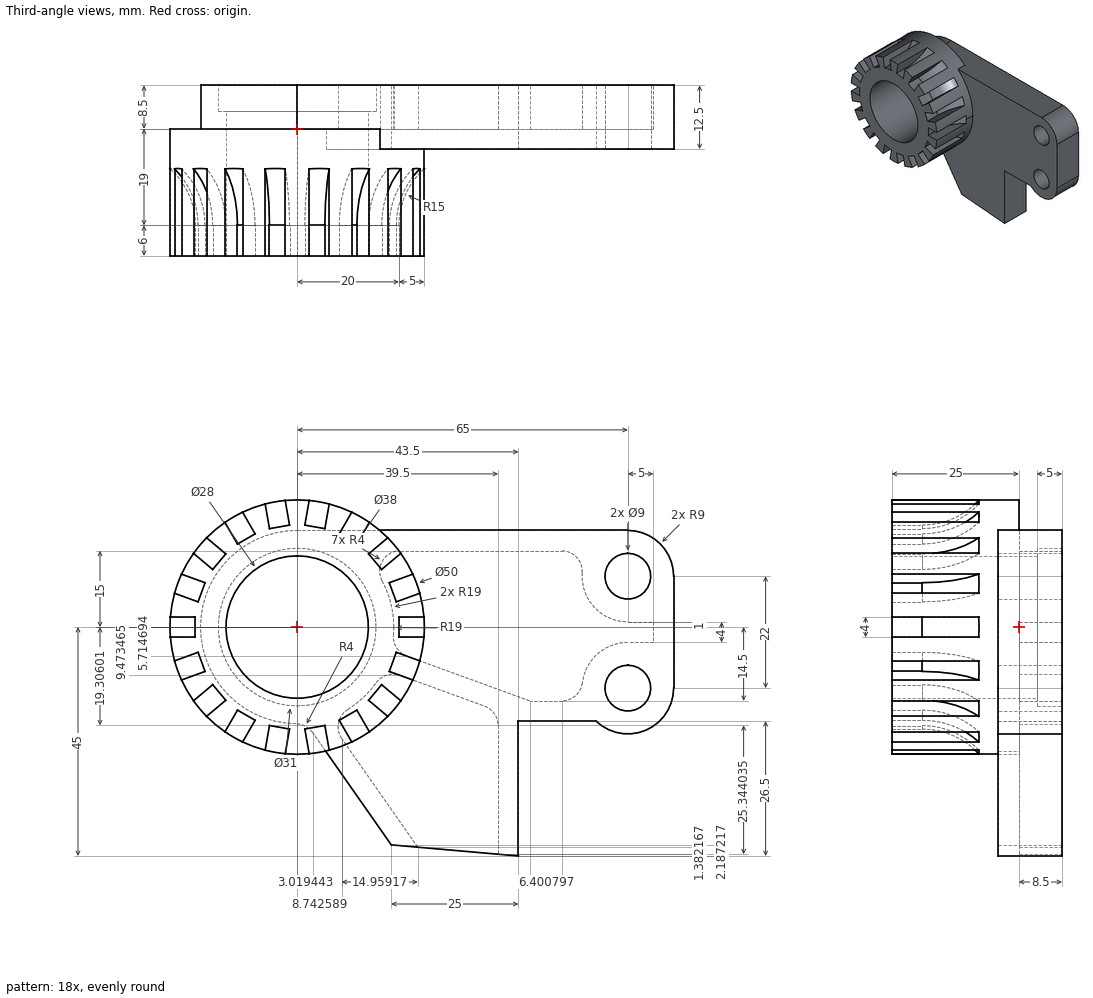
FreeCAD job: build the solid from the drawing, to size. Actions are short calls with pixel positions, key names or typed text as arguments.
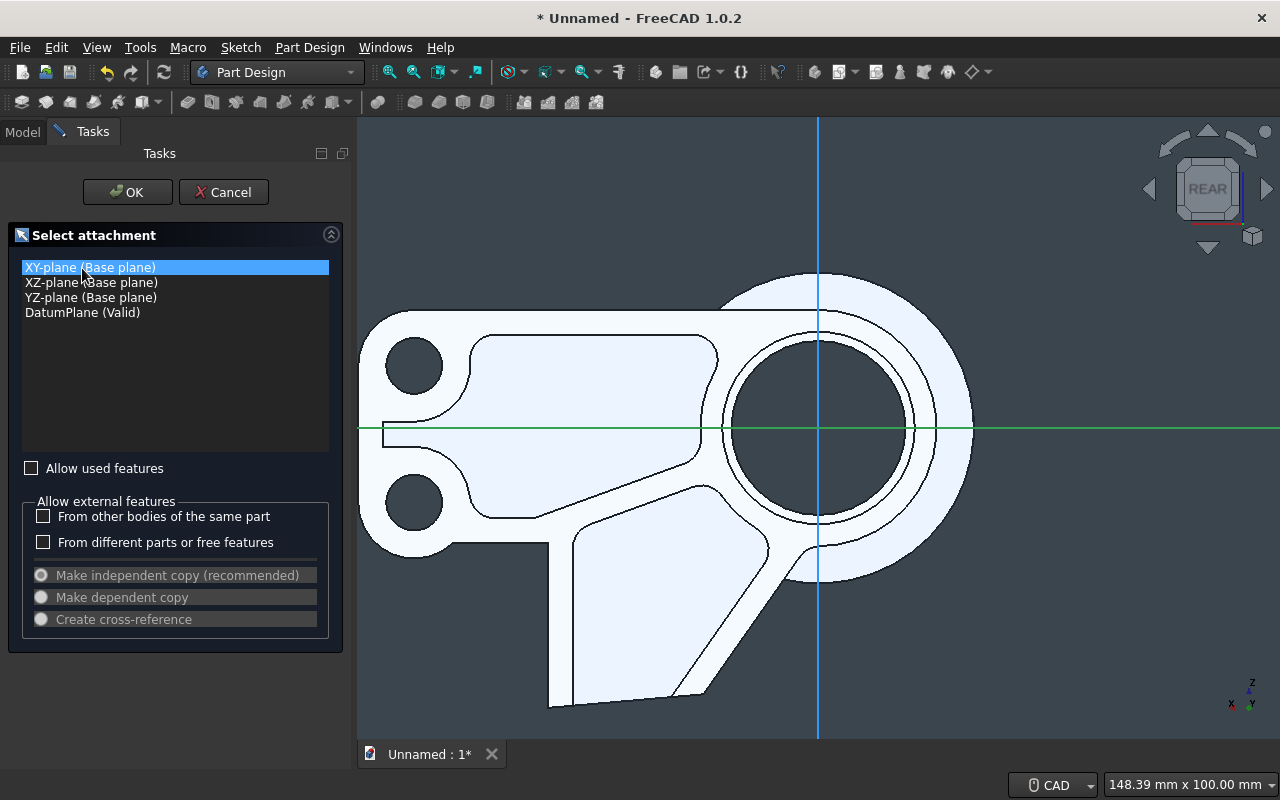
click(128, 192)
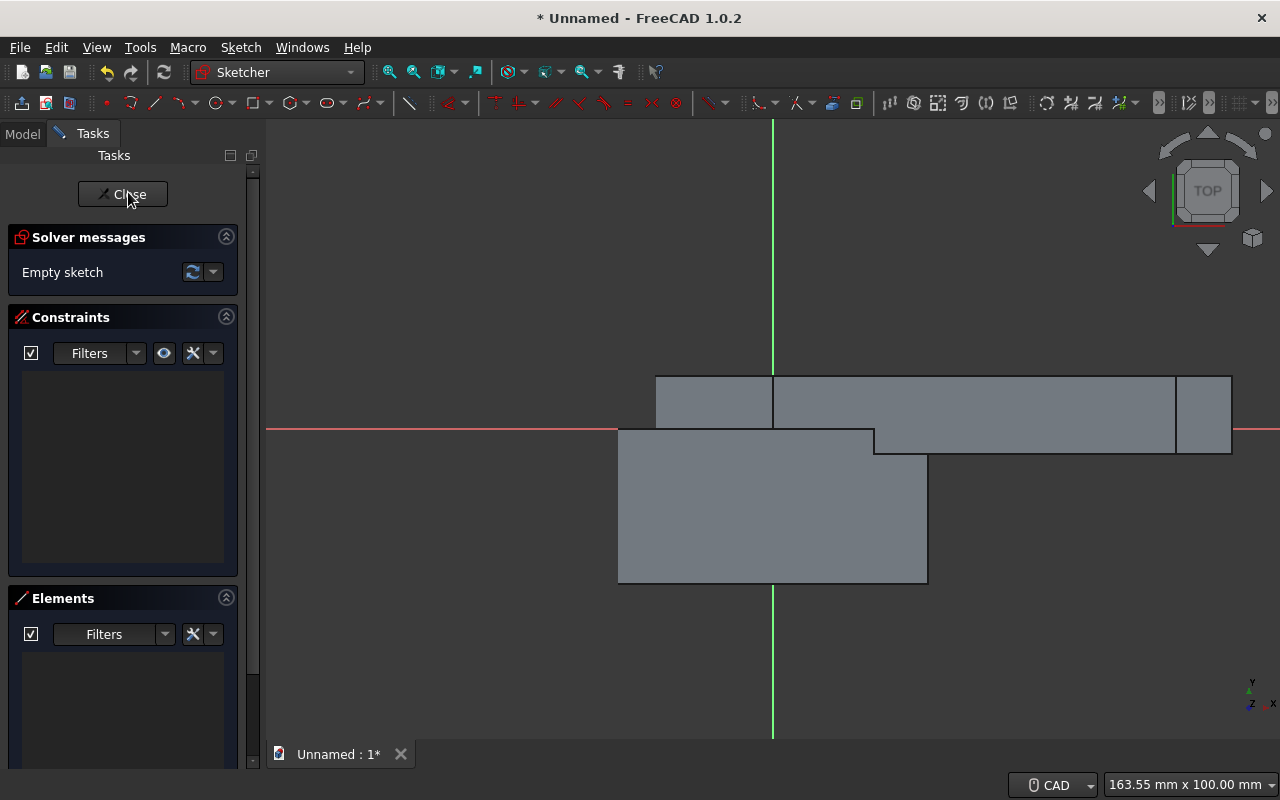
click(70, 104)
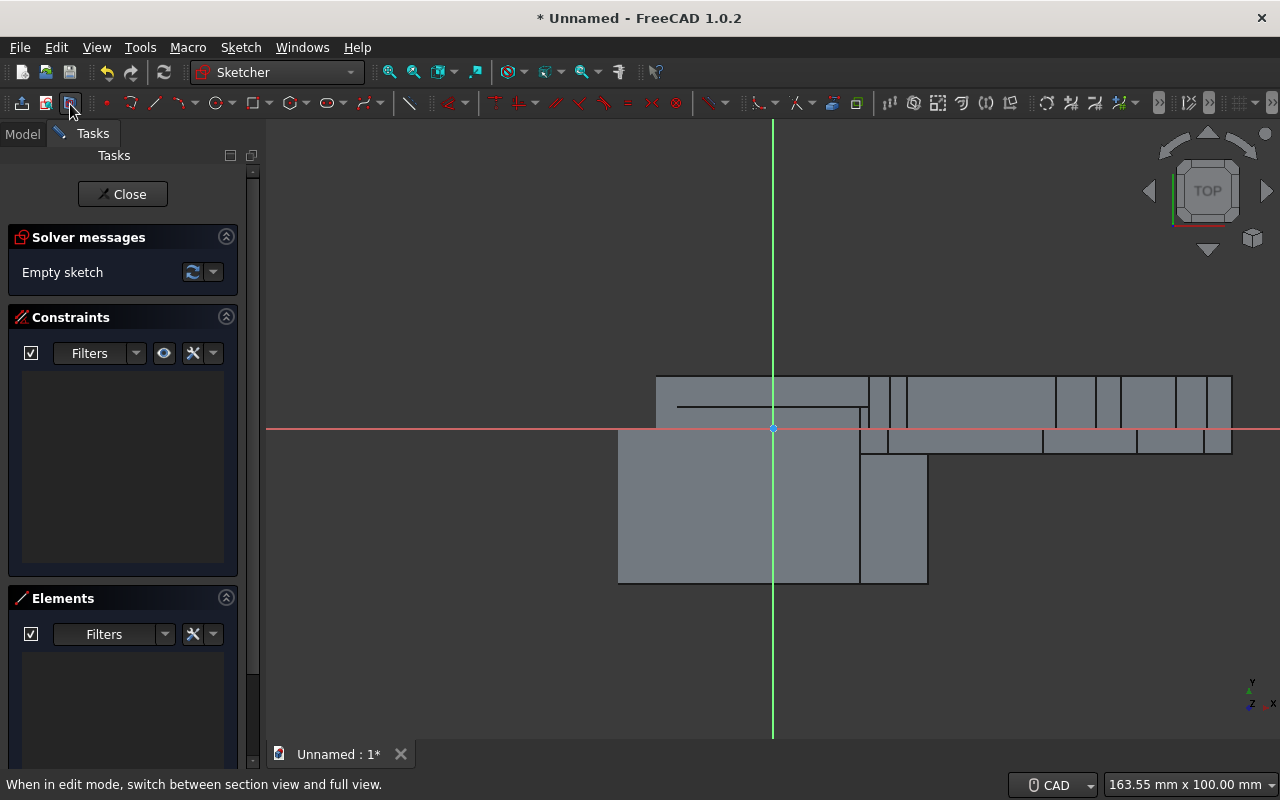
scroll(935, 552, up, 5)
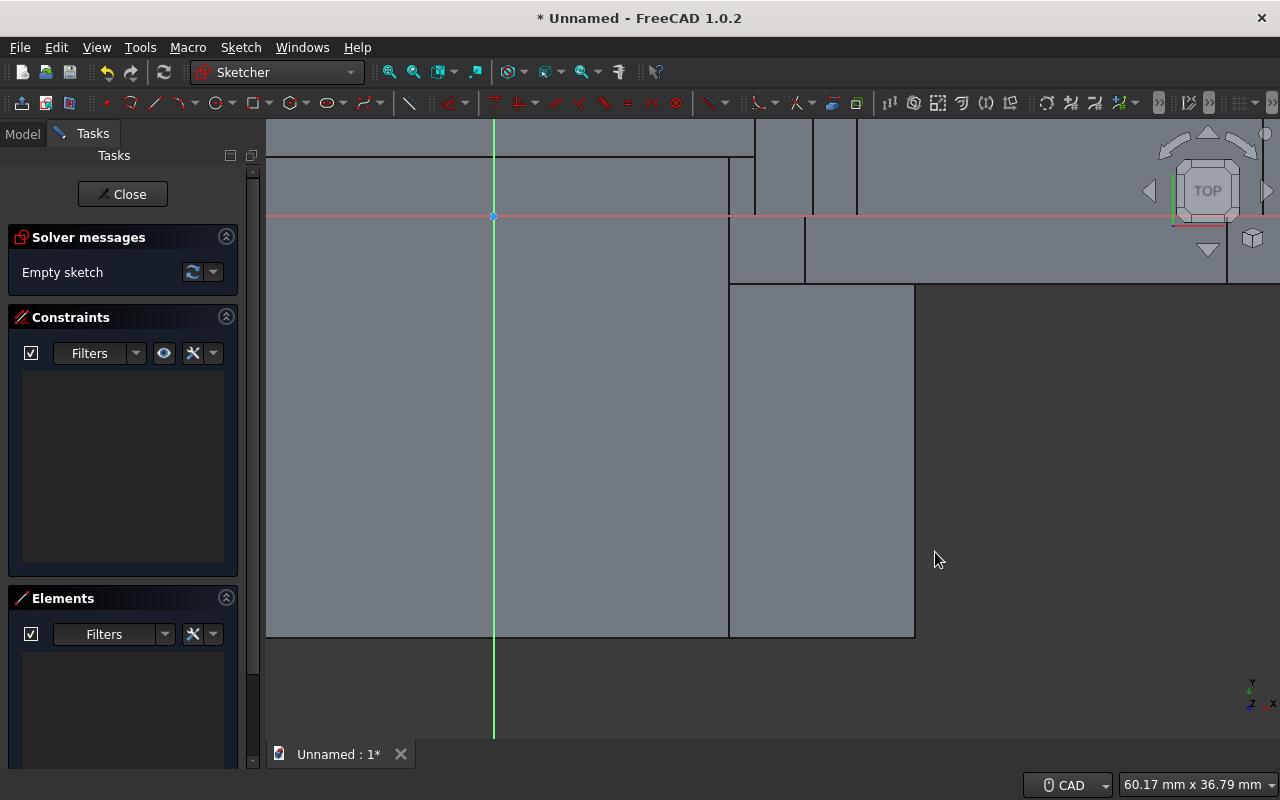
click(132, 104)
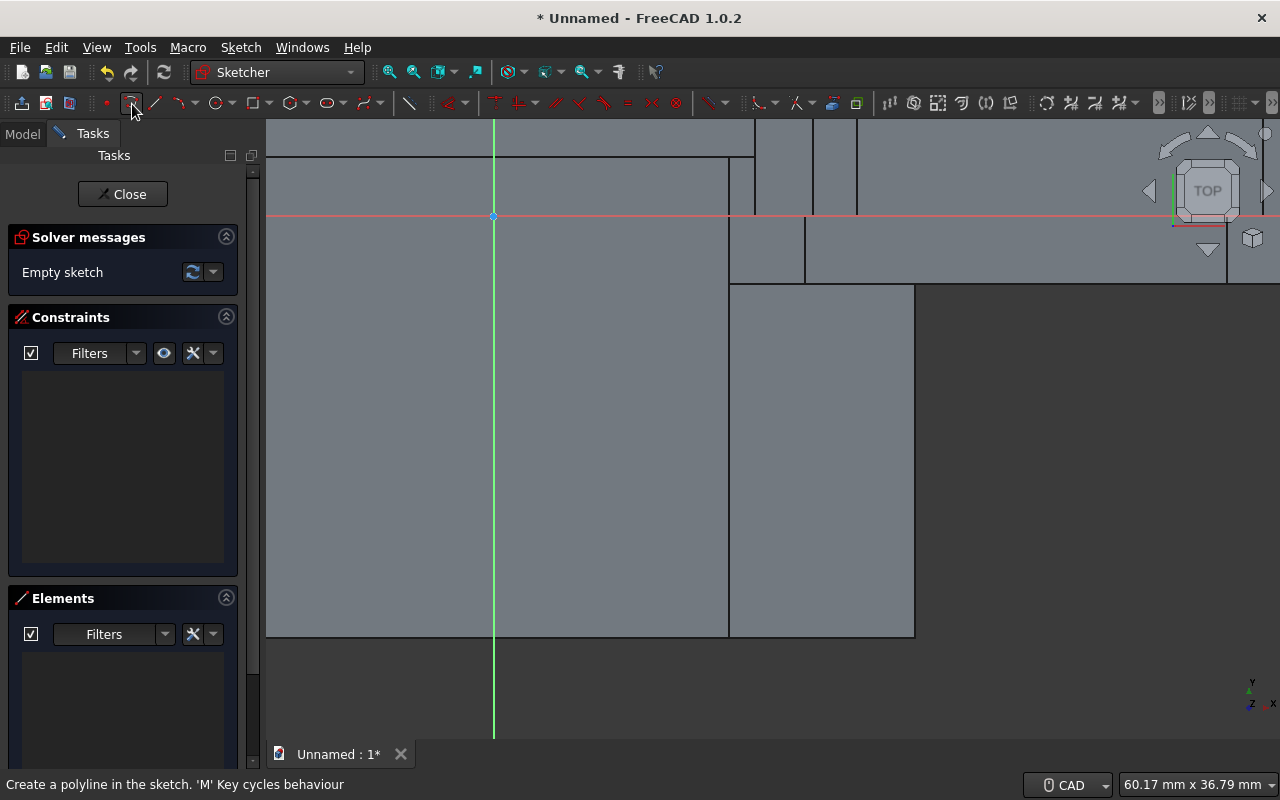
click(831, 537)
click(831, 638)
click(915, 638)
click(915, 348)
right_click(915, 348)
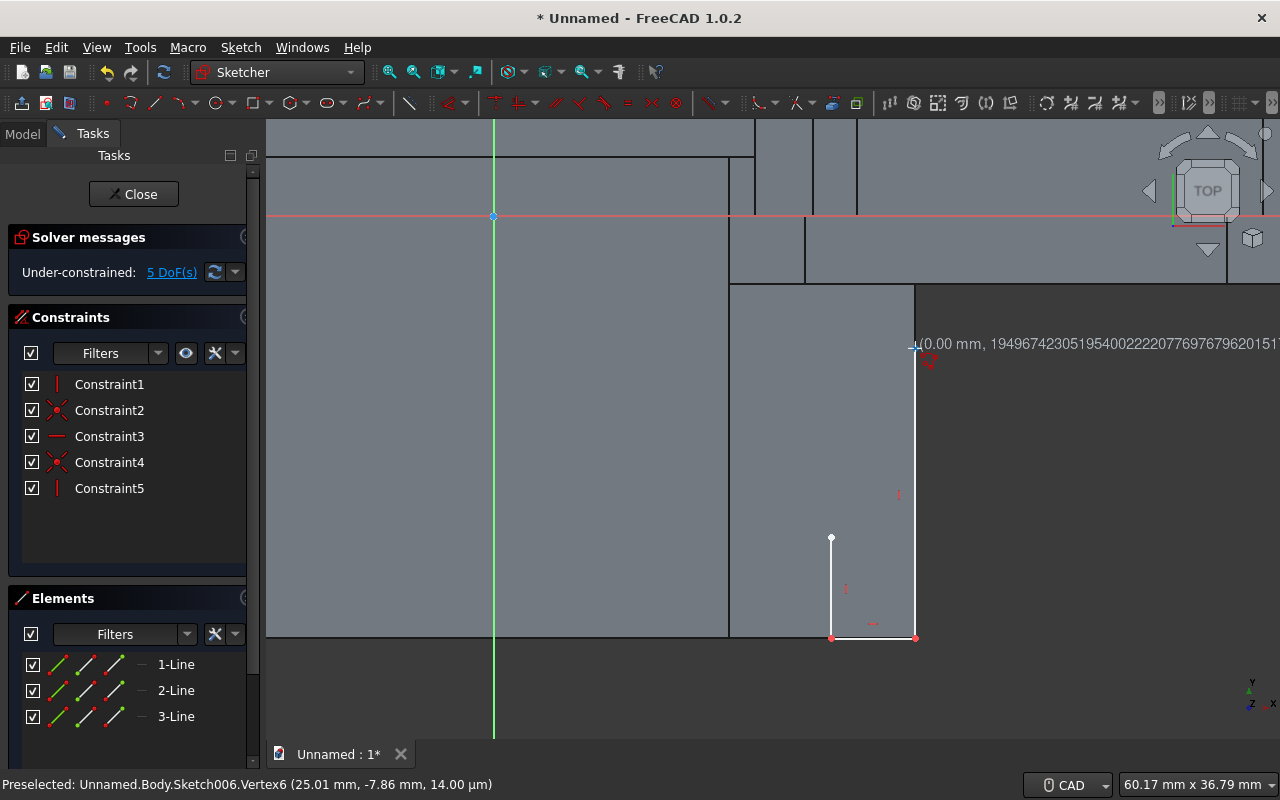
click(180, 104)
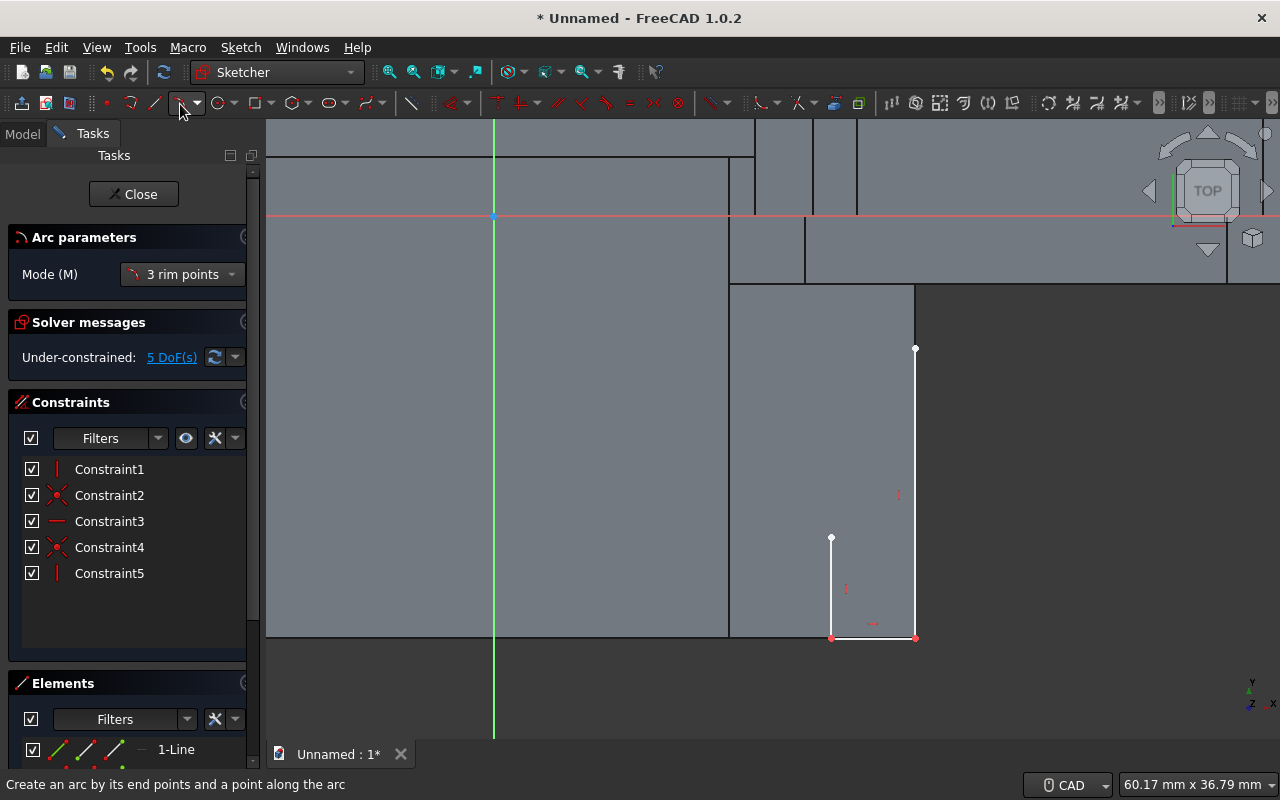
click(915, 349)
click(831, 538)
click(853, 433)
key(Escape)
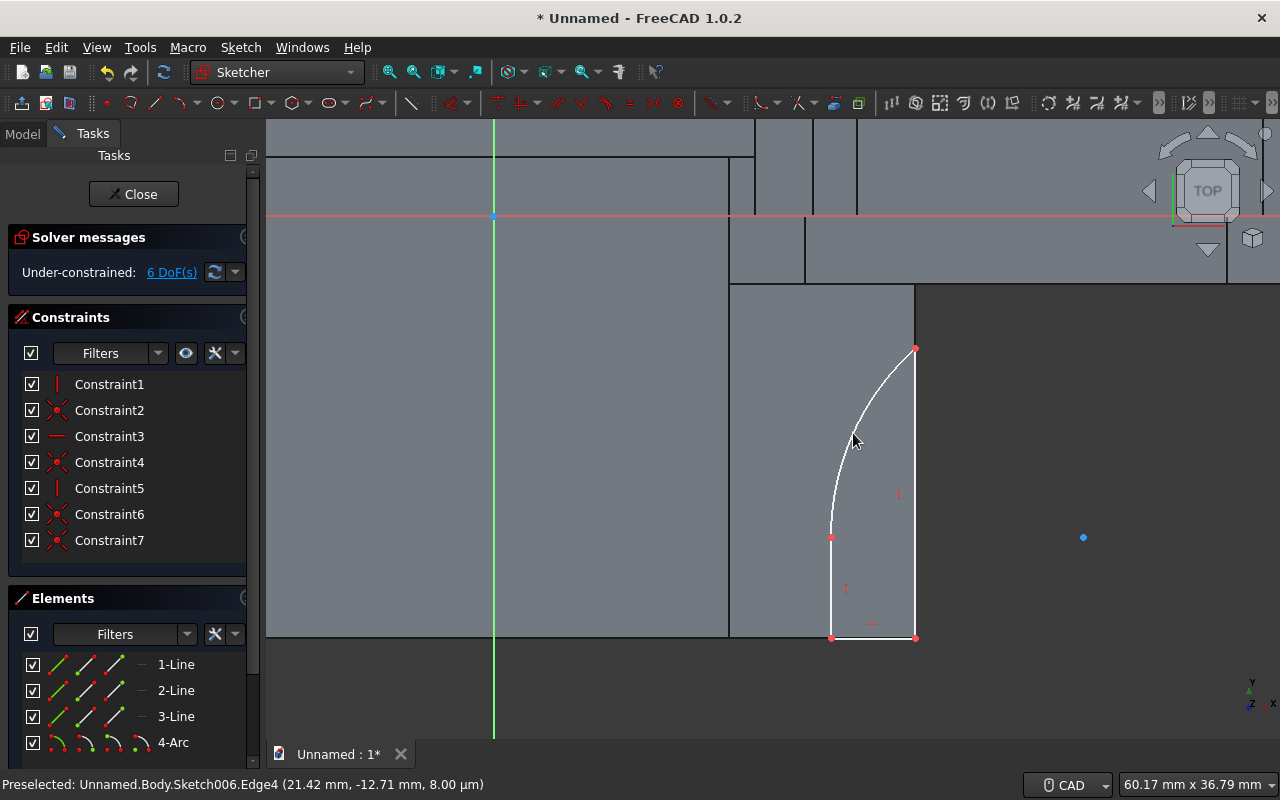
click(831, 568)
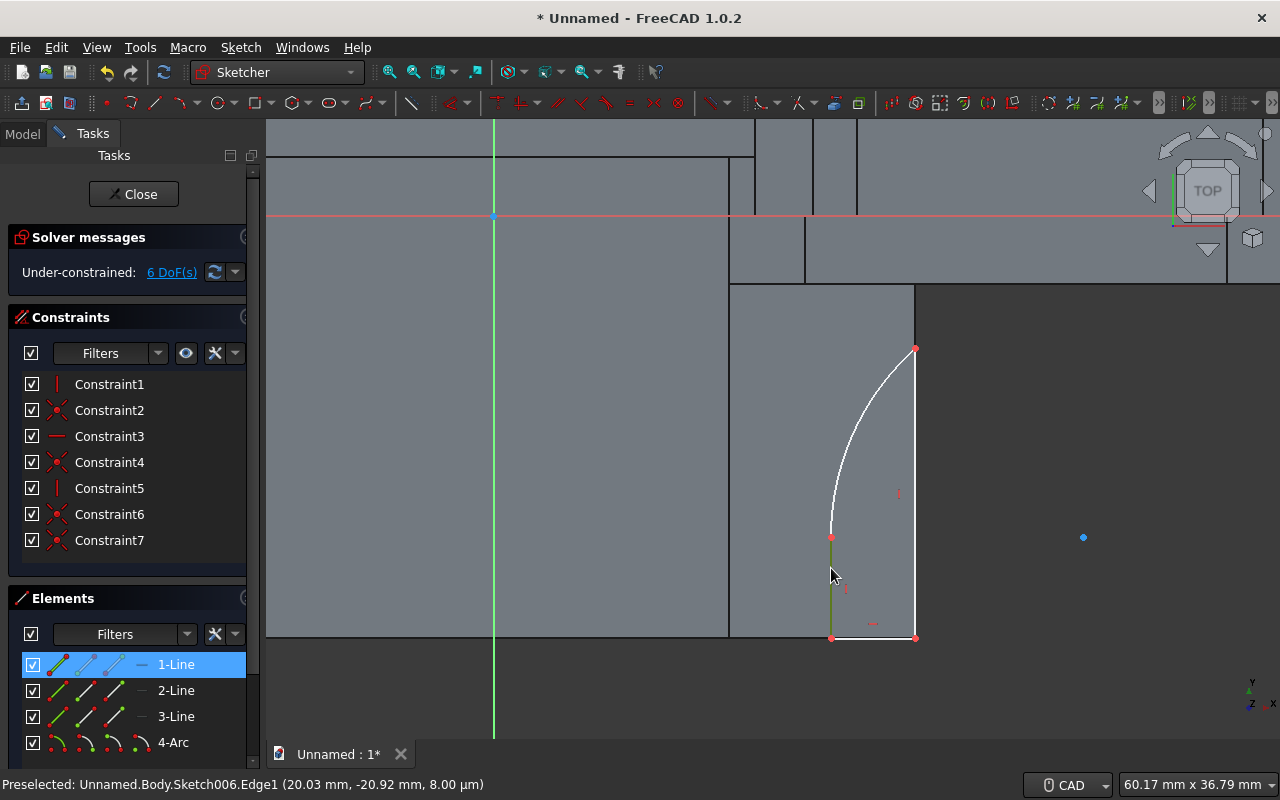
click(873, 397)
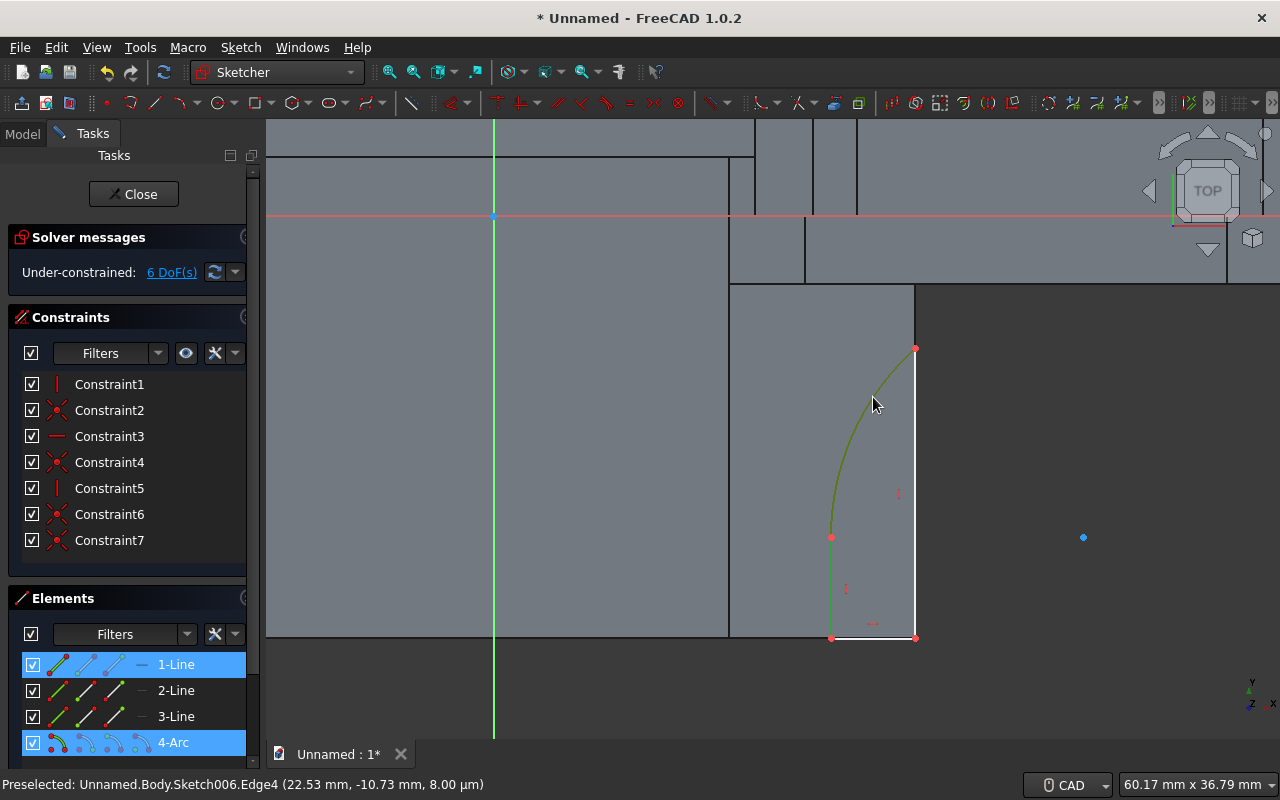
click(606, 104)